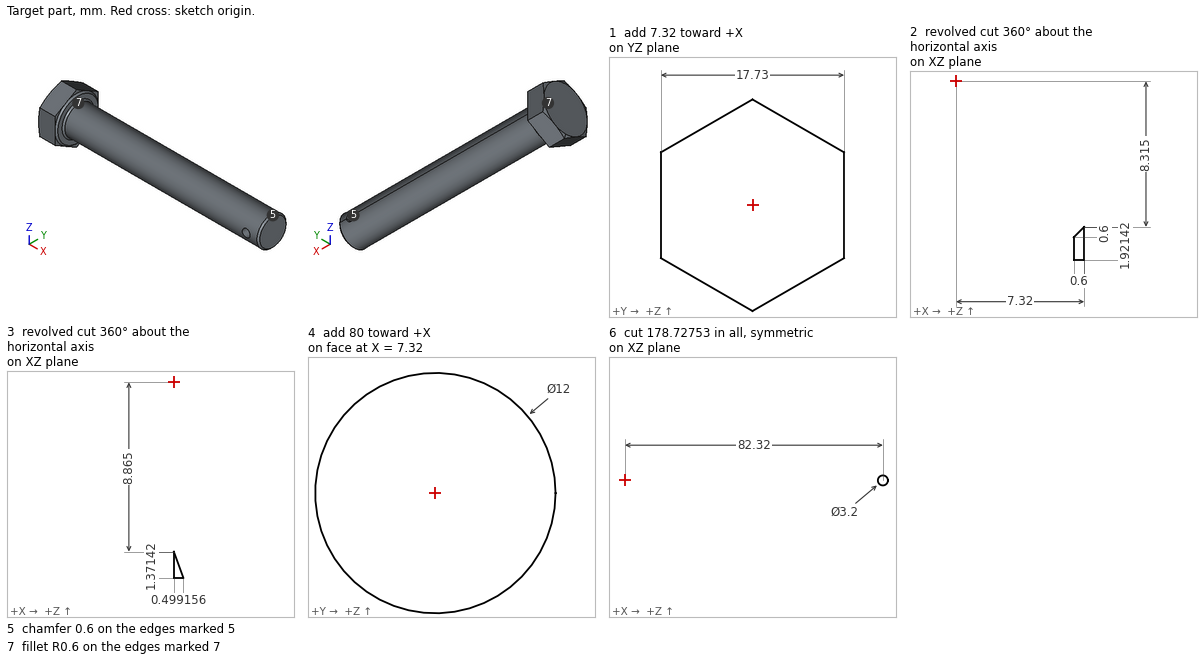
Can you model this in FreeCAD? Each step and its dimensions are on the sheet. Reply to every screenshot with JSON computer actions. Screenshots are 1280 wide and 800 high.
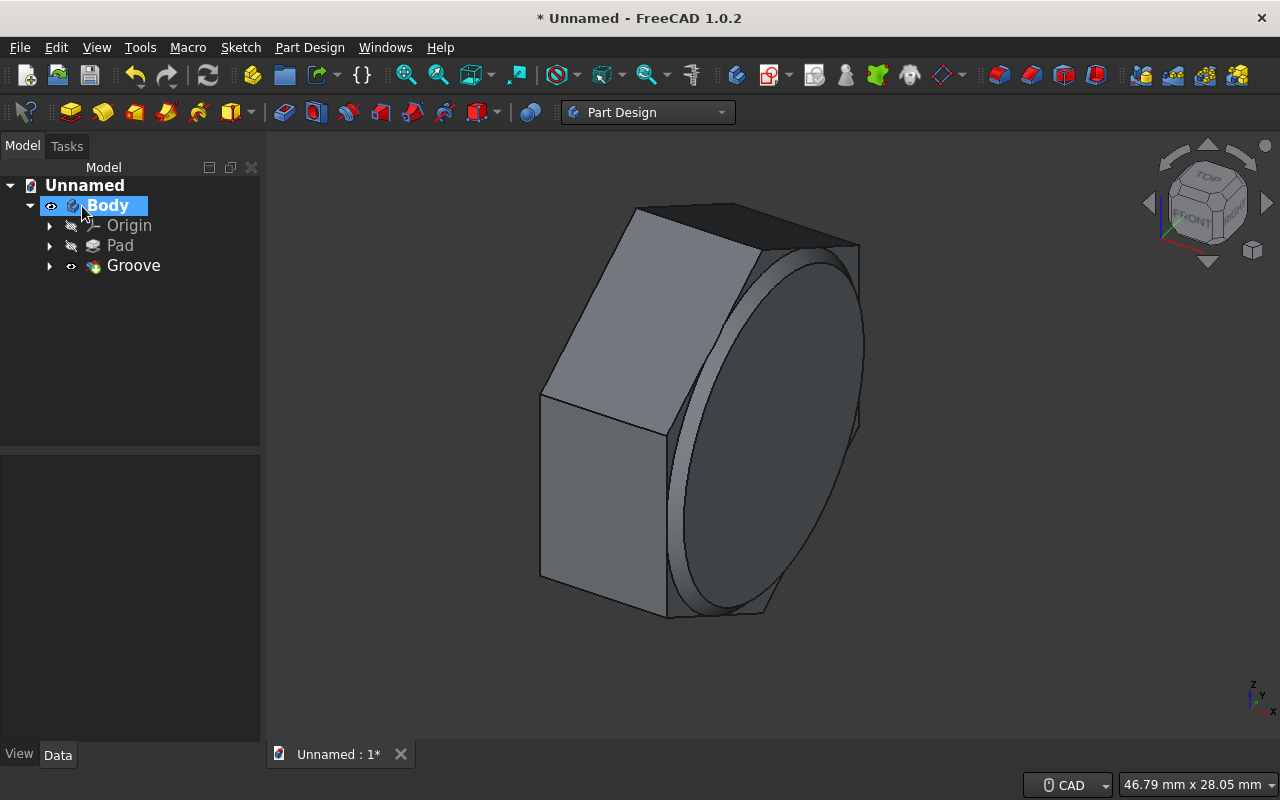
{"action": "left_click", "coordinate": [408, 76]}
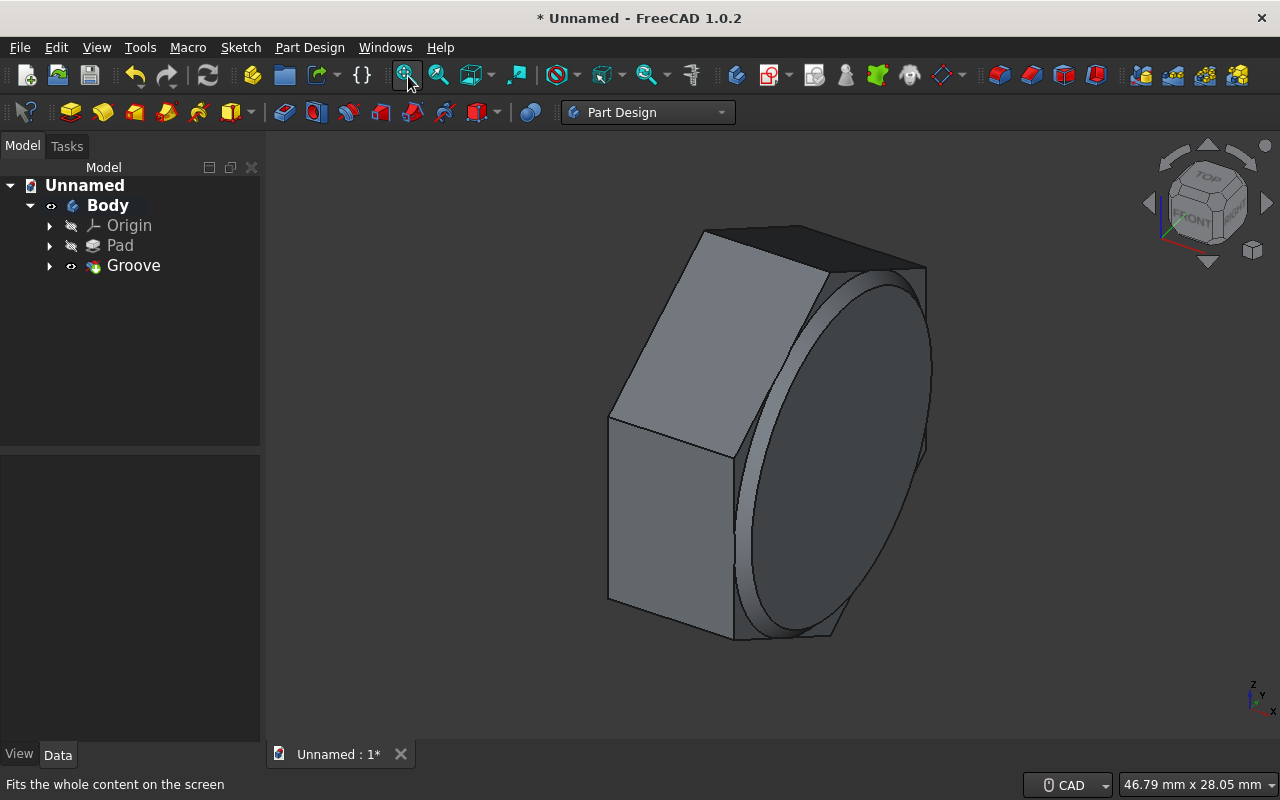
{"action": "left_click", "coordinate": [770, 76]}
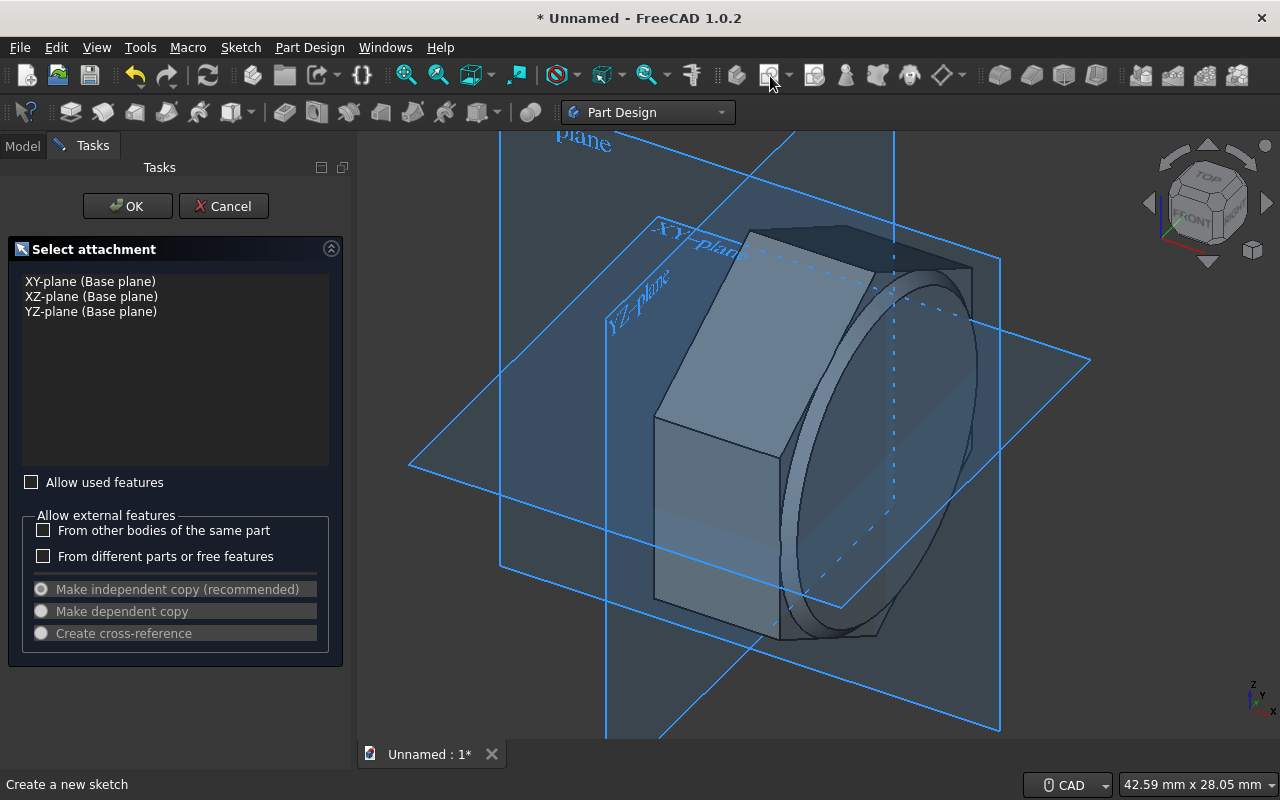
{"action": "left_click", "coordinate": [82, 296]}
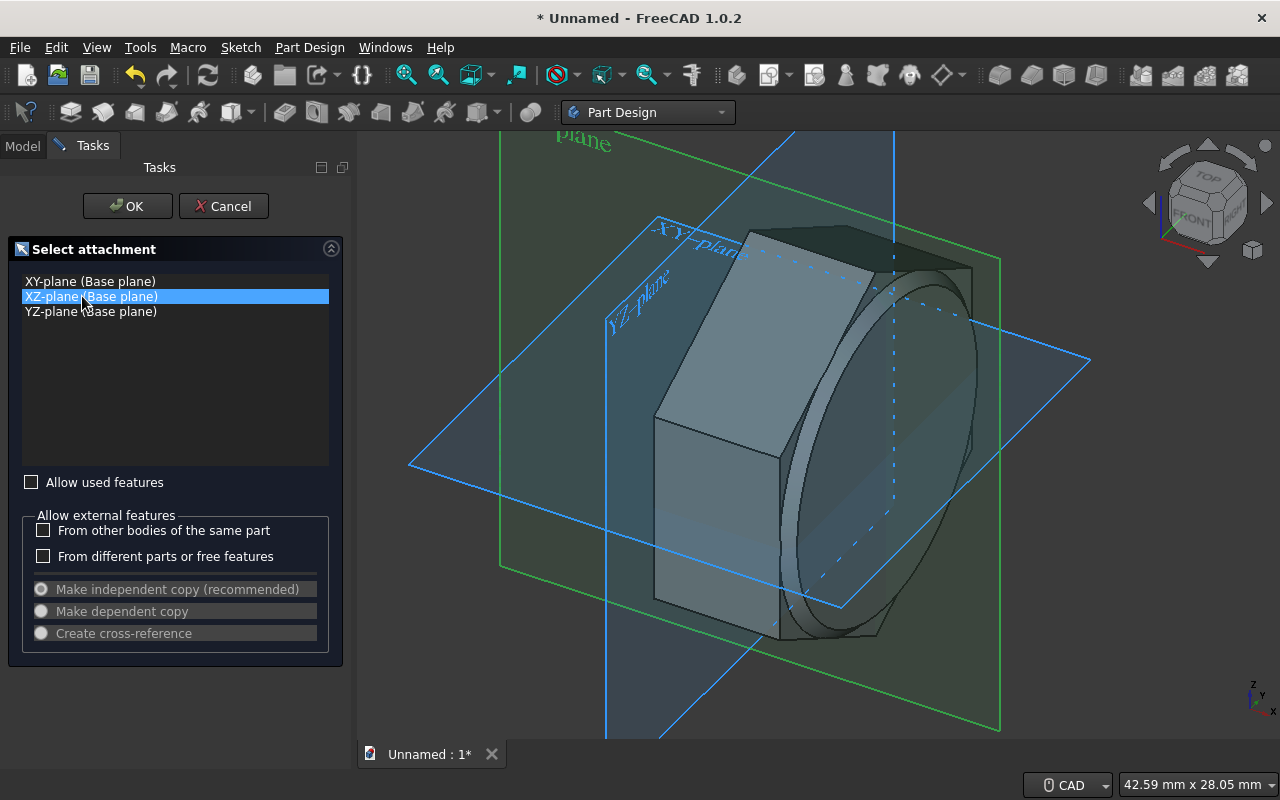
{"action": "left_click", "coordinate": [128, 206]}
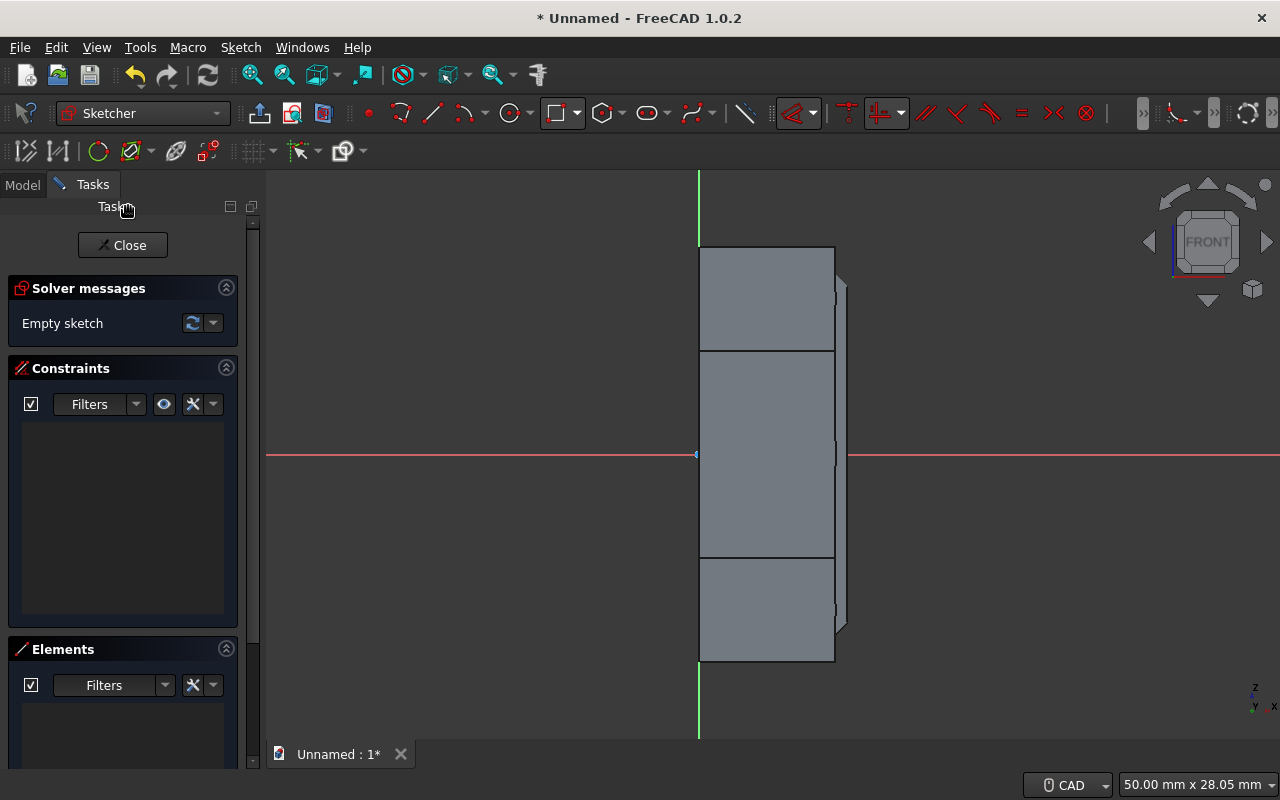
{"action": "left_click", "coordinate": [324, 114]}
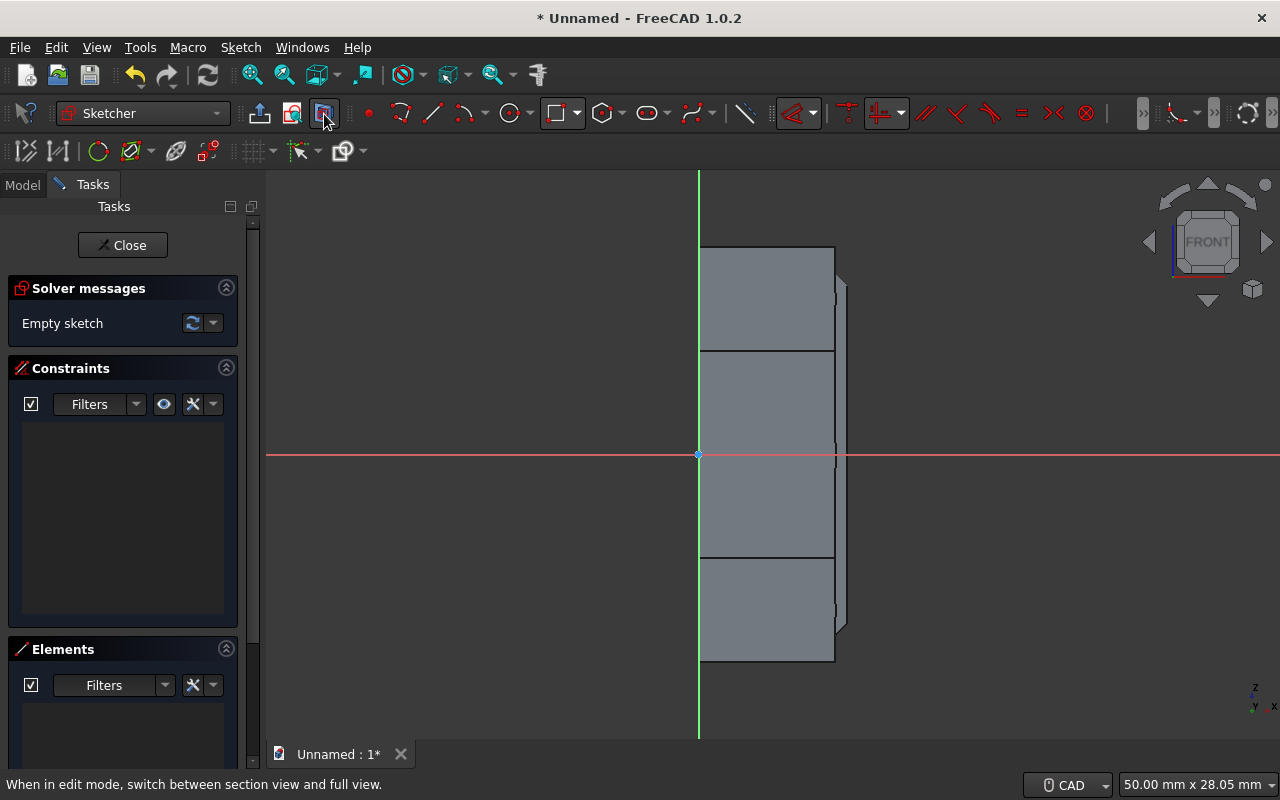
{"action": "scroll", "coordinate": [704, 664], "scroll_direction": "up", "scroll_amount": 13}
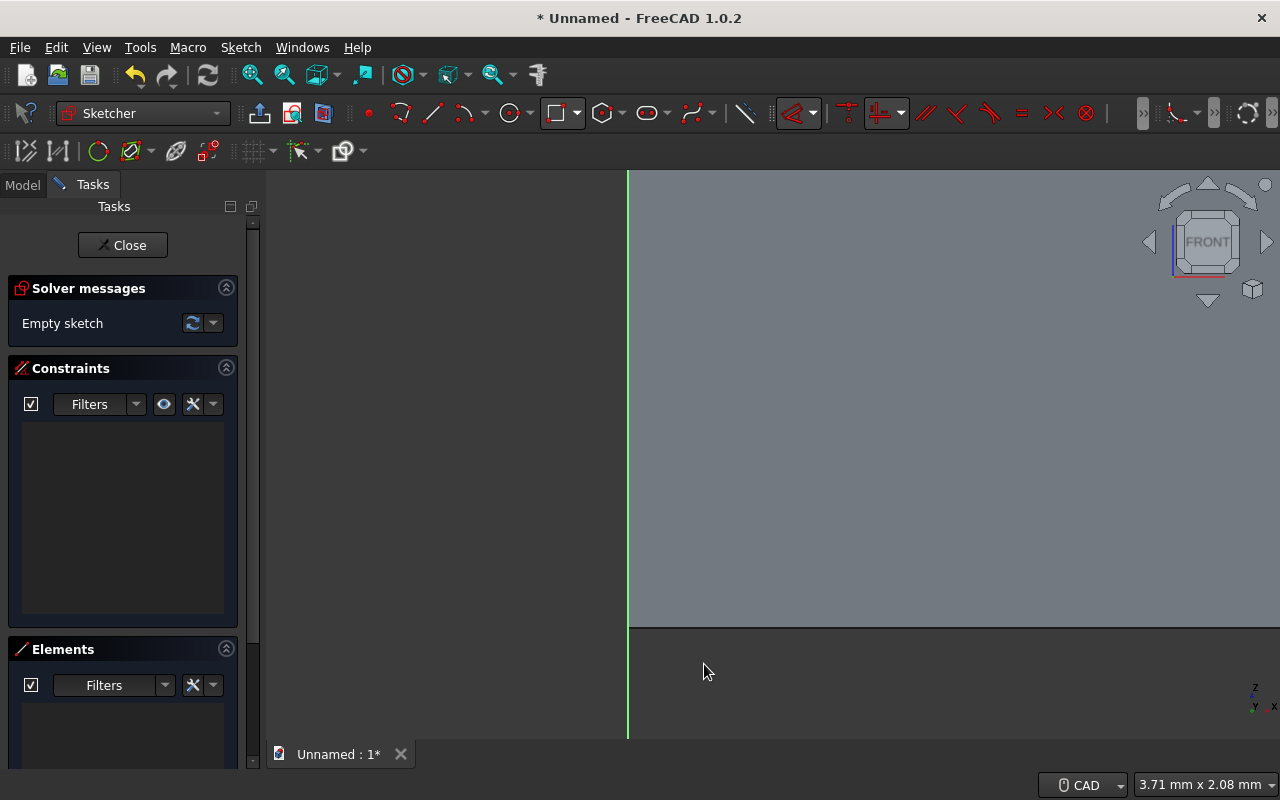
{"action": "left_click", "coordinate": [402, 114]}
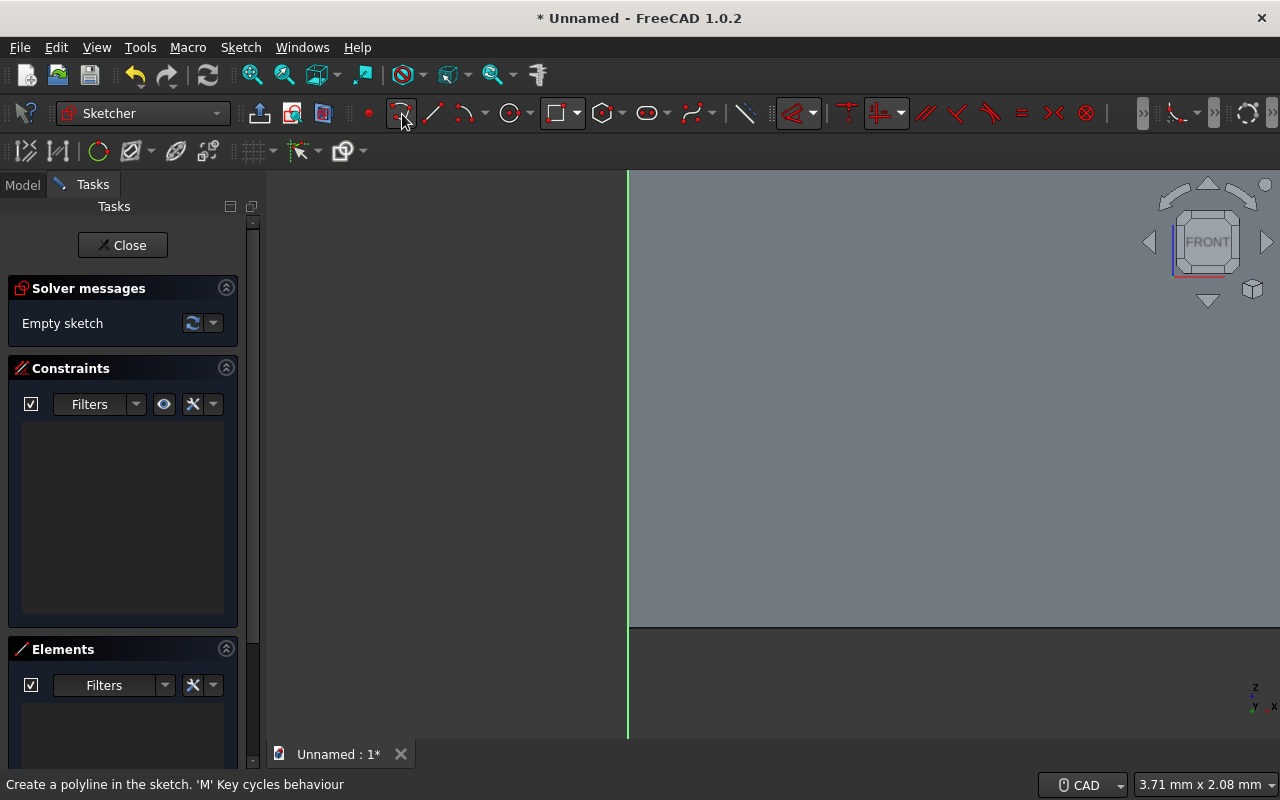
{"action": "left_click", "coordinate": [628, 253]}
{"action": "left_click", "coordinate": [764, 628]}
{"action": "left_click", "coordinate": [637, 628]}
{"action": "left_click", "coordinate": [628, 254]}
{"action": "key", "text": "Escape"}
{"action": "key", "text": "Escape"}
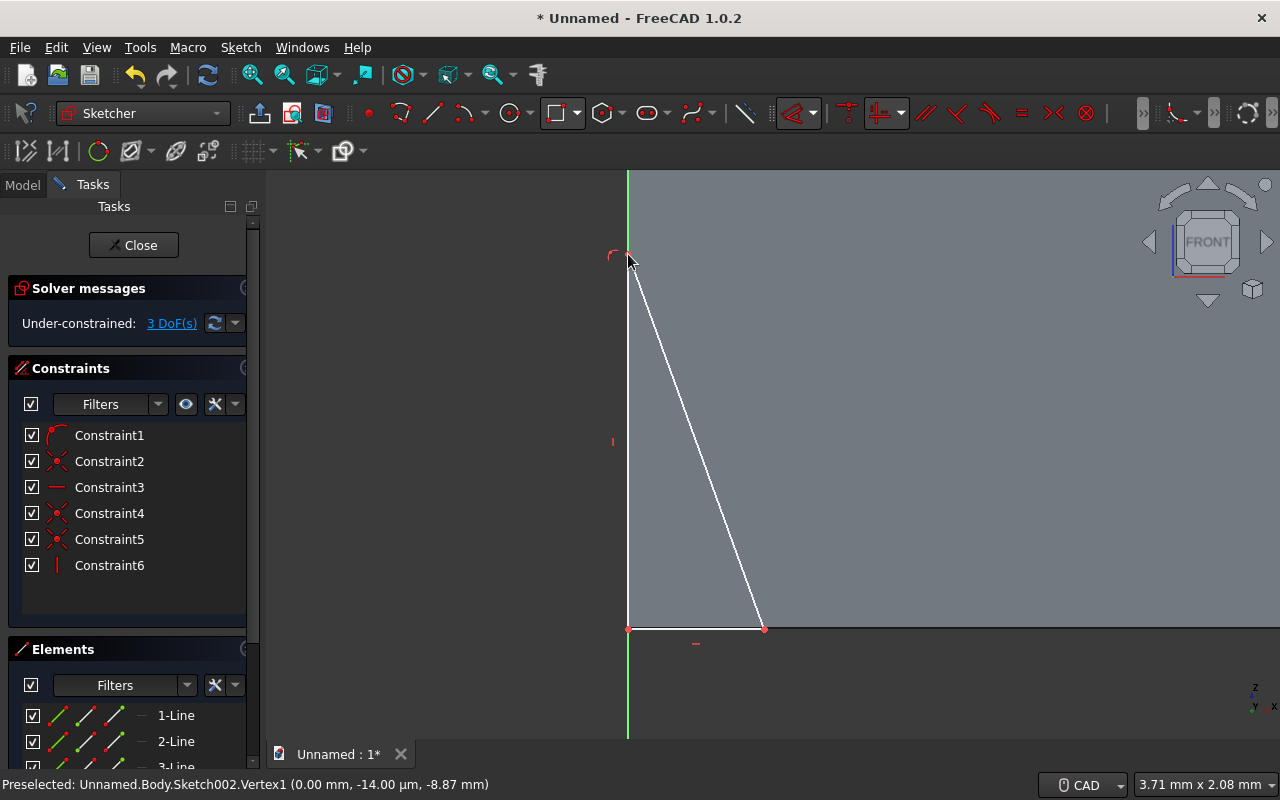
{"action": "left_click", "coordinate": [628, 254]}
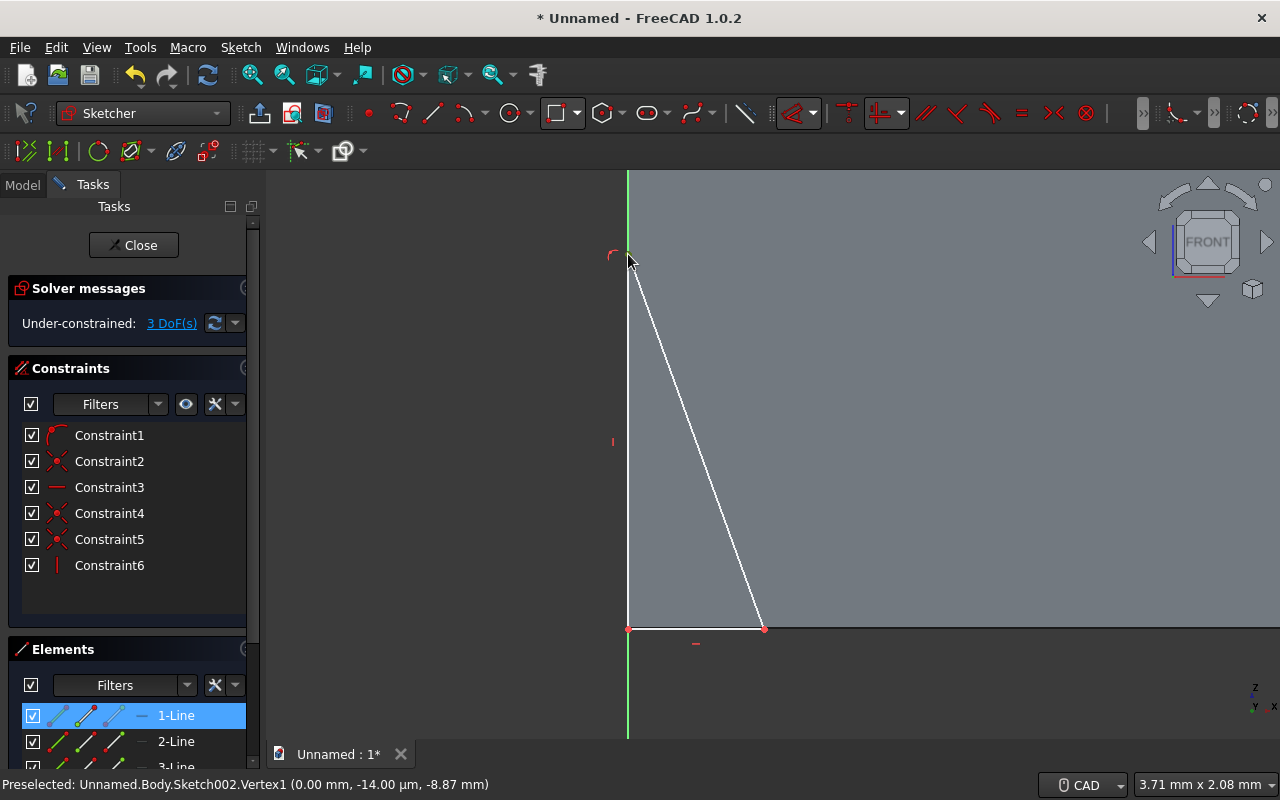
{"action": "key", "text": "i"}